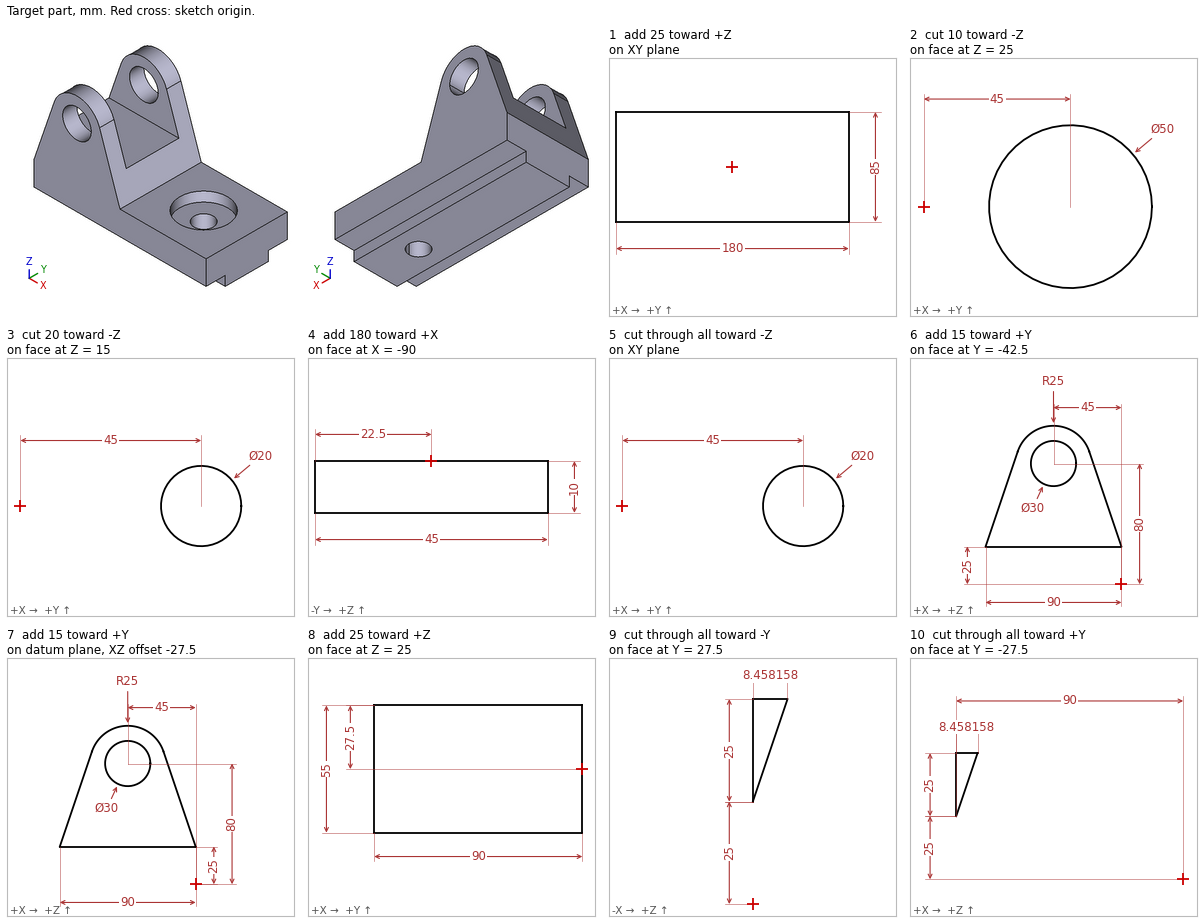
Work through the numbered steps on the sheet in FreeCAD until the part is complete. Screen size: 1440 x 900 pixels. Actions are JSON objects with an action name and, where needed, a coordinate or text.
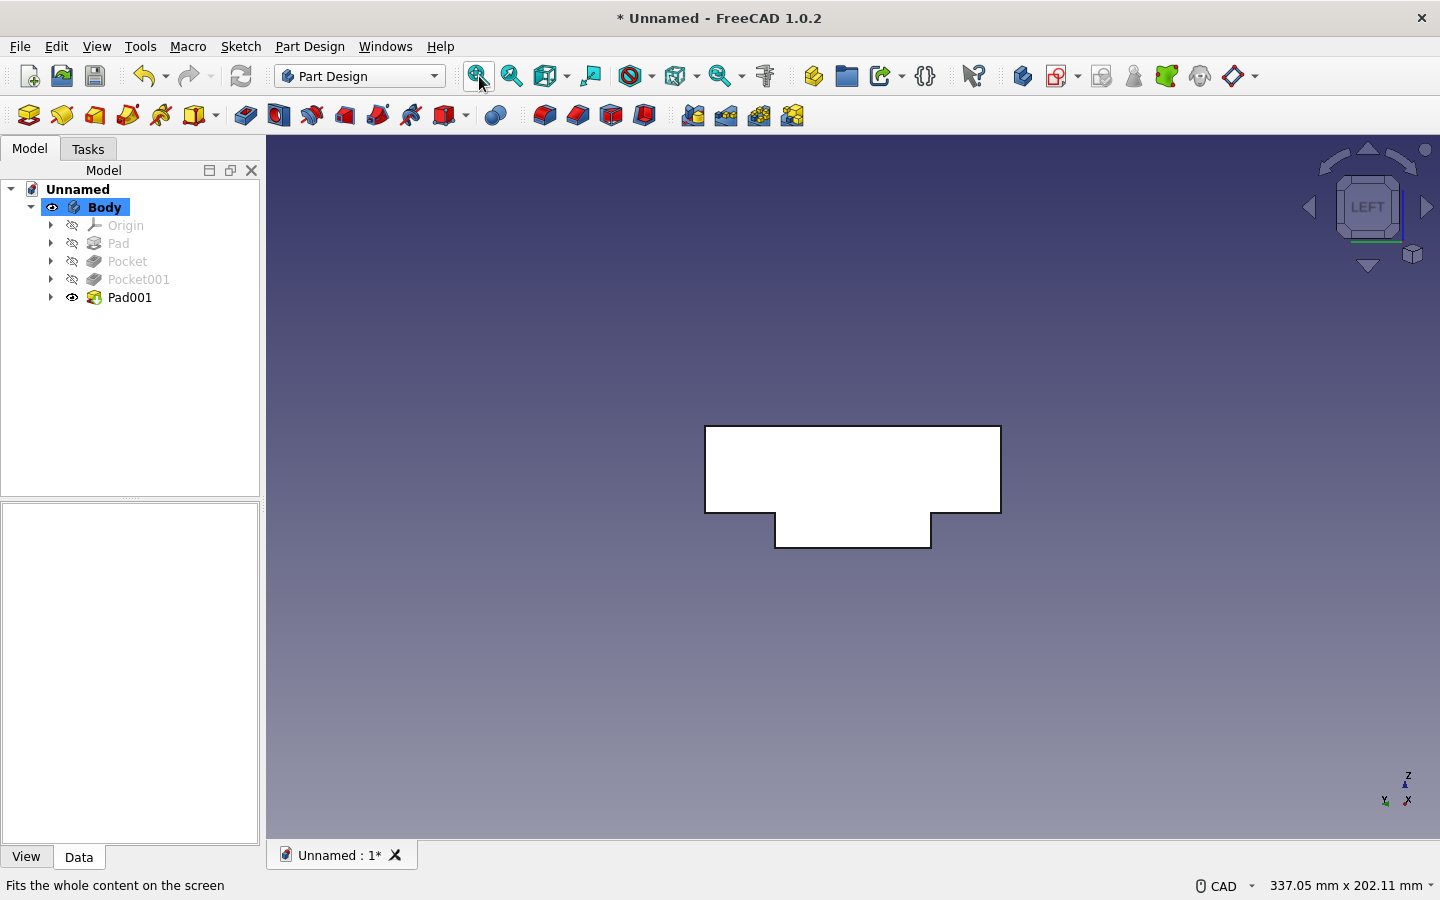
{"action": "left_click", "coordinate": [1056, 76]}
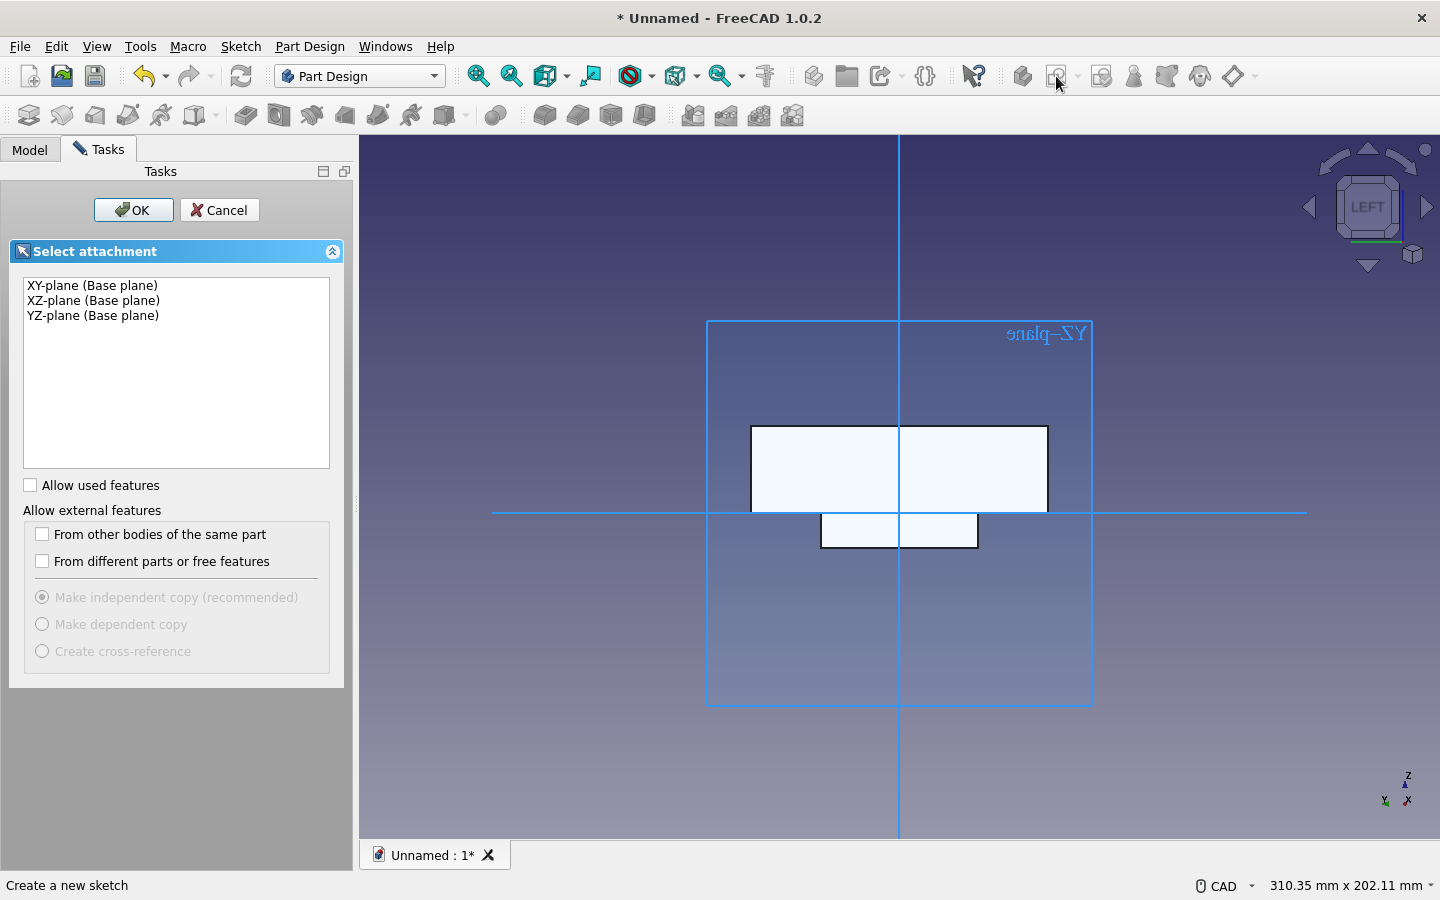
{"action": "left_click", "coordinate": [84, 286]}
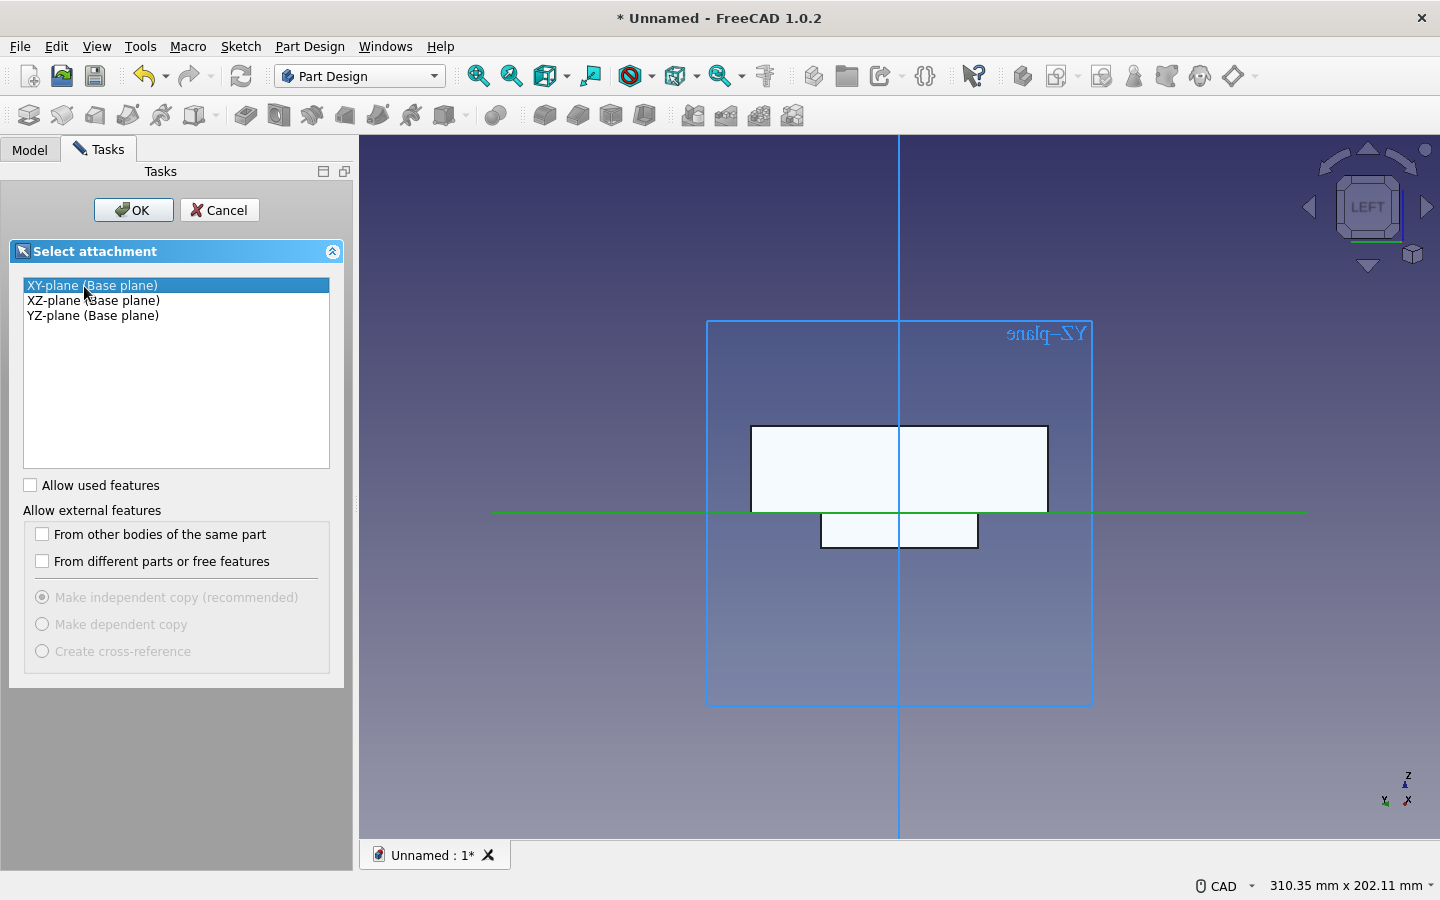
{"action": "left_click", "coordinate": [134, 210]}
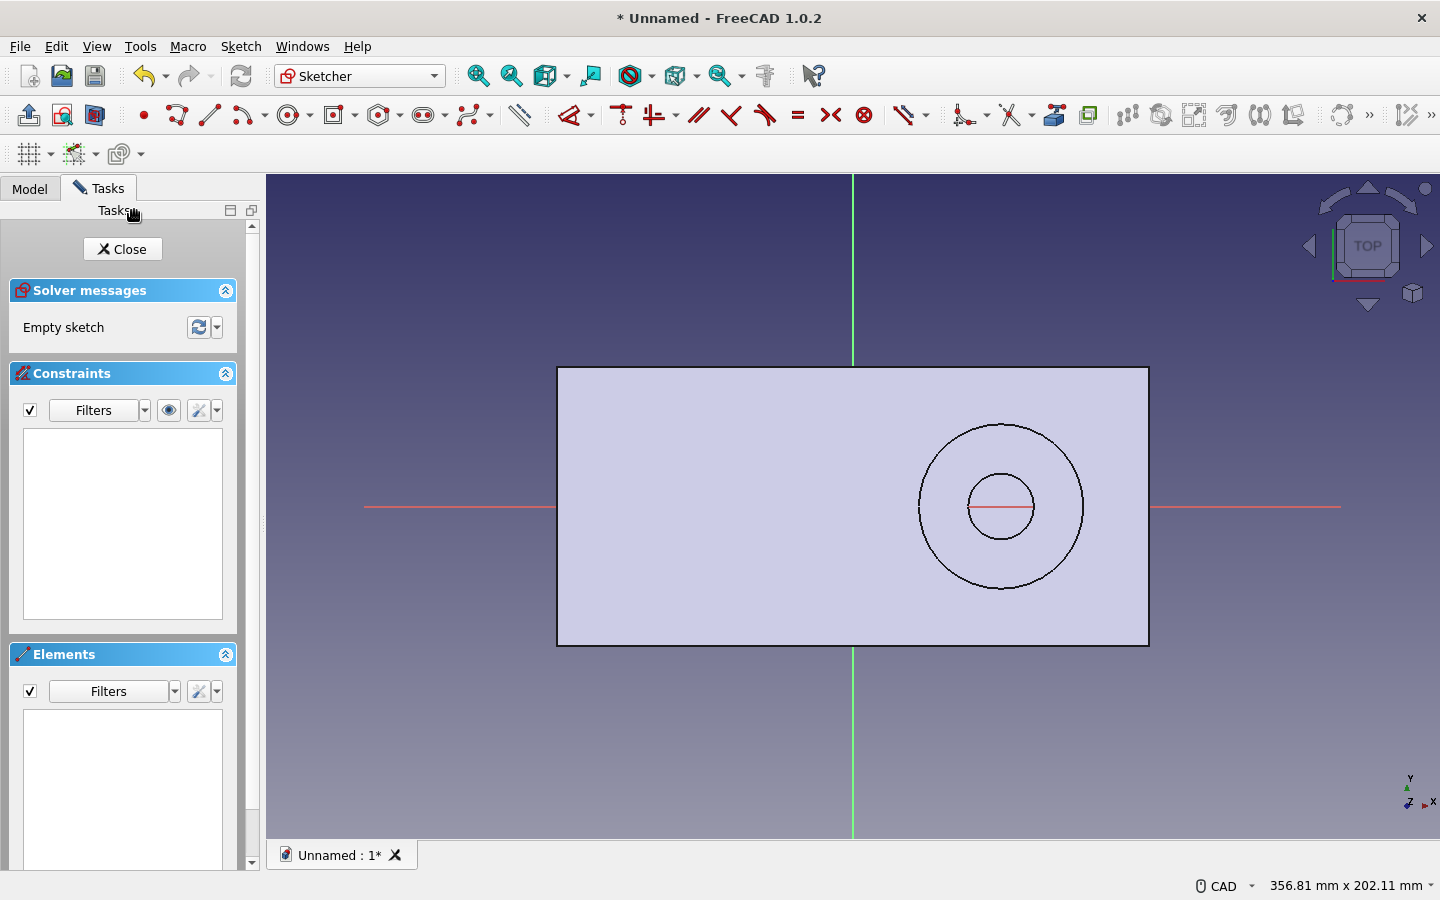
{"action": "left_click", "coordinate": [95, 116]}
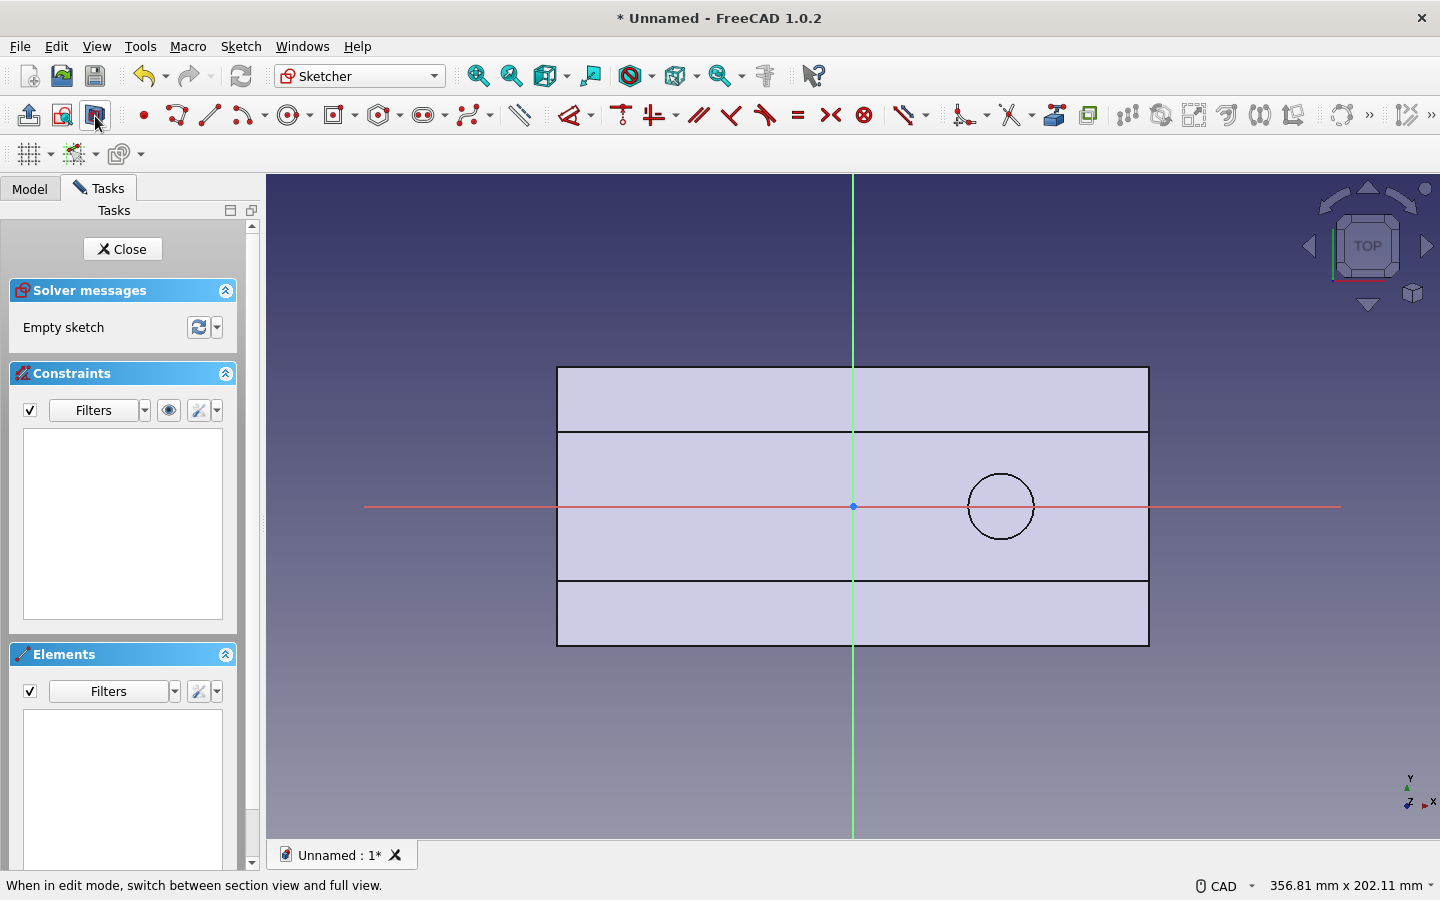
{"action": "scroll", "coordinate": [1044, 506], "scroll_direction": "up", "scroll_amount": 9}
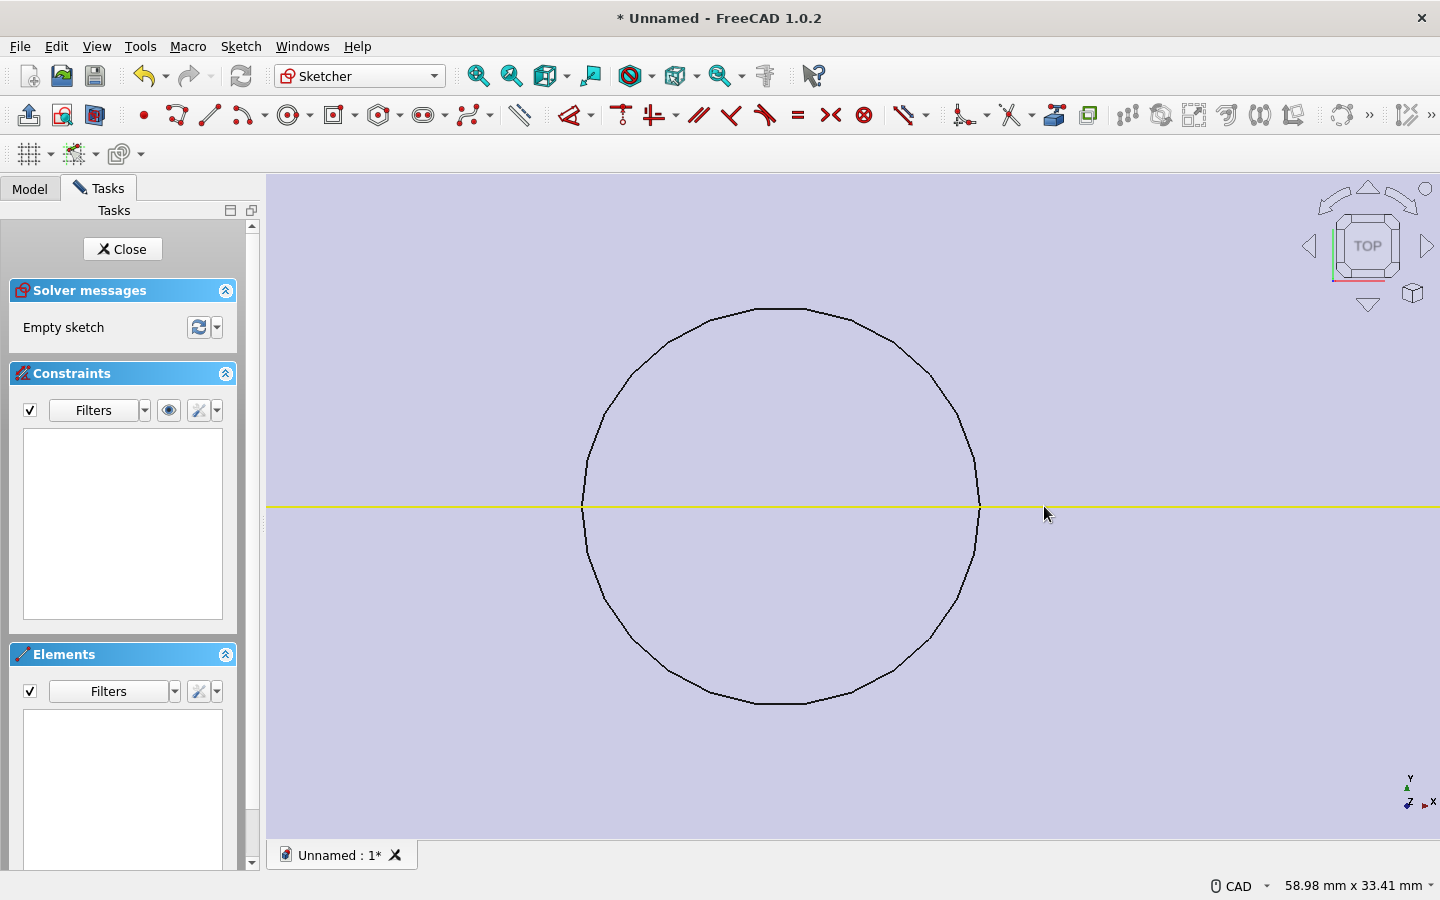
{"action": "left_click", "coordinate": [288, 116]}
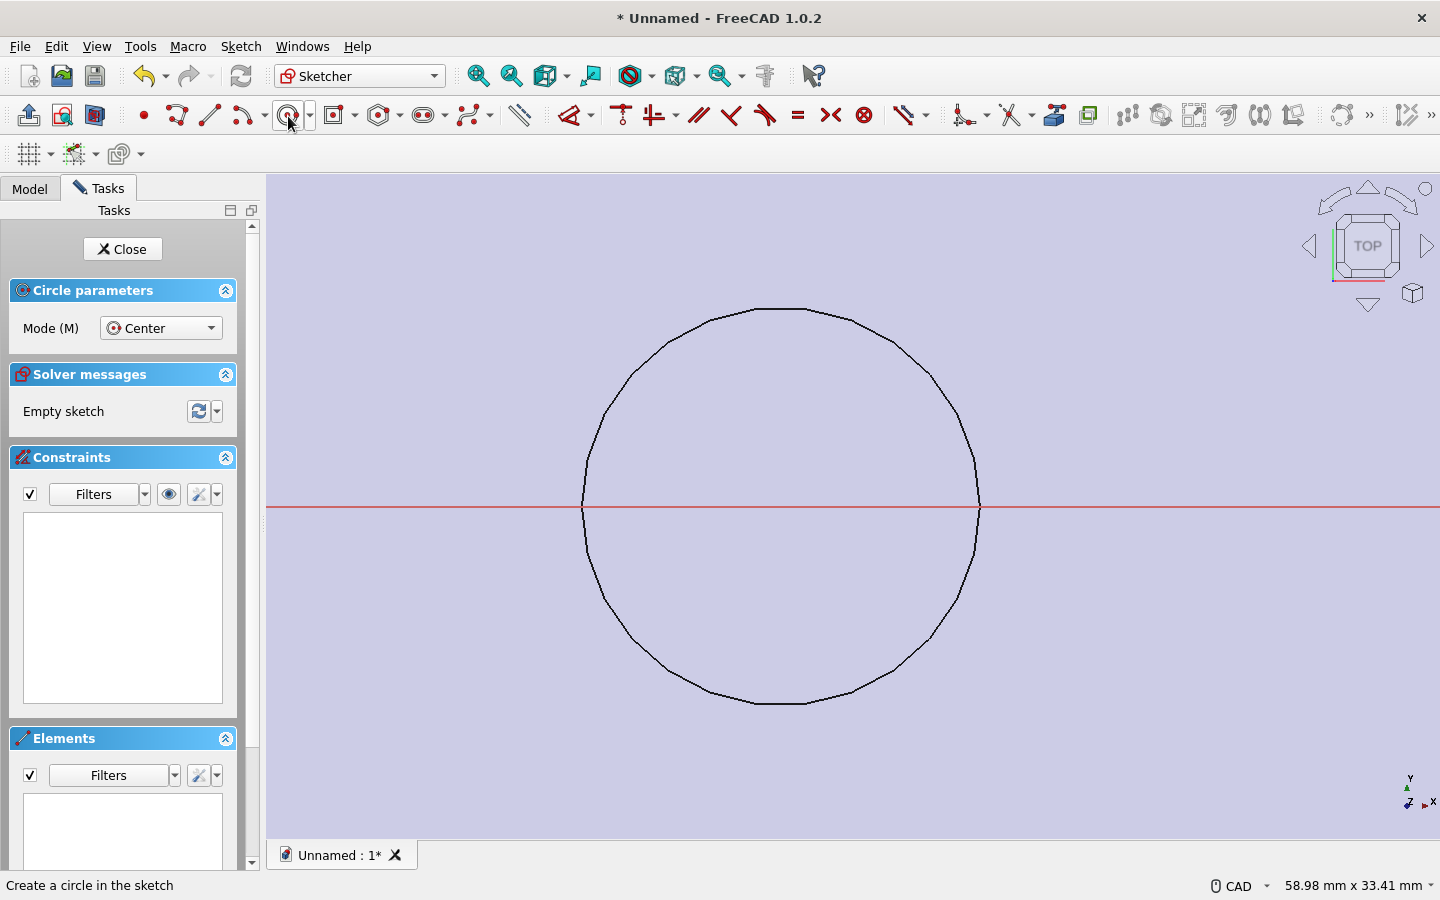
{"action": "left_click", "coordinate": [781, 506]}
{"action": "mouse_move", "coordinate": [922, 366]}